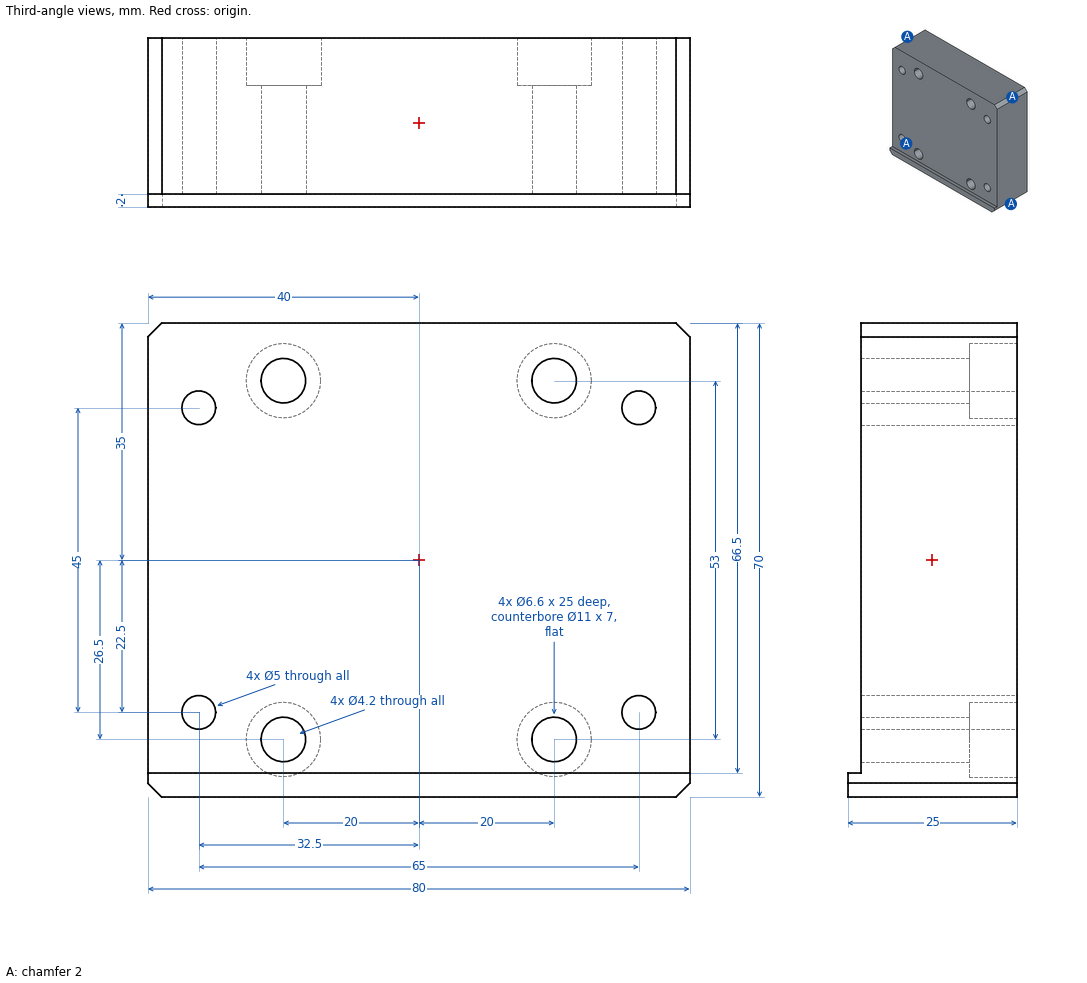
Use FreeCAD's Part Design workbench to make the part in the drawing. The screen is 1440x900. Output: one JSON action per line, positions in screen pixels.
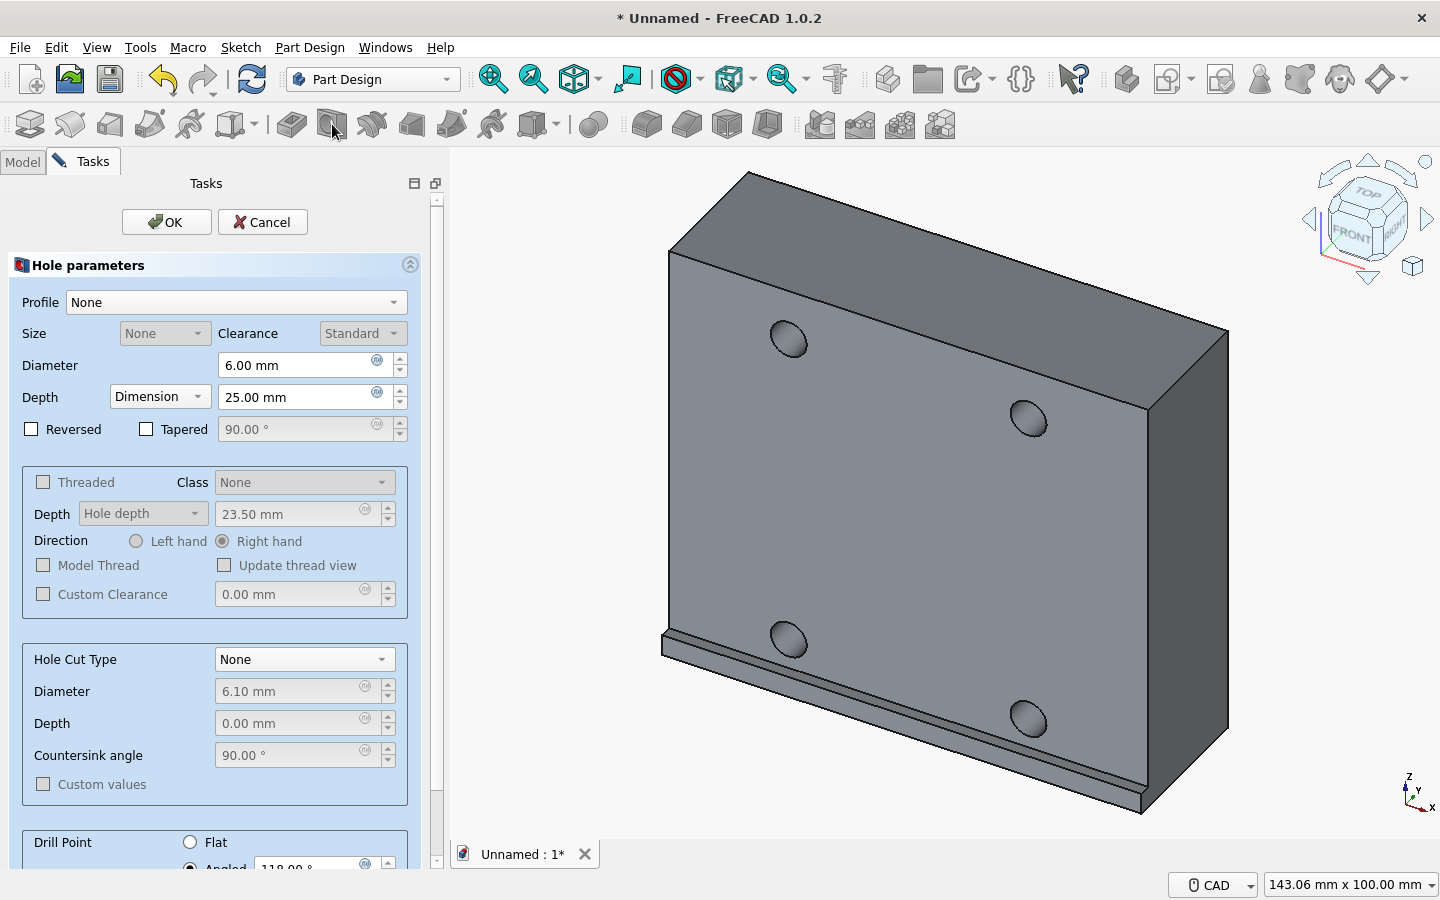
{"action": "triple_click", "coordinate": [305, 365]}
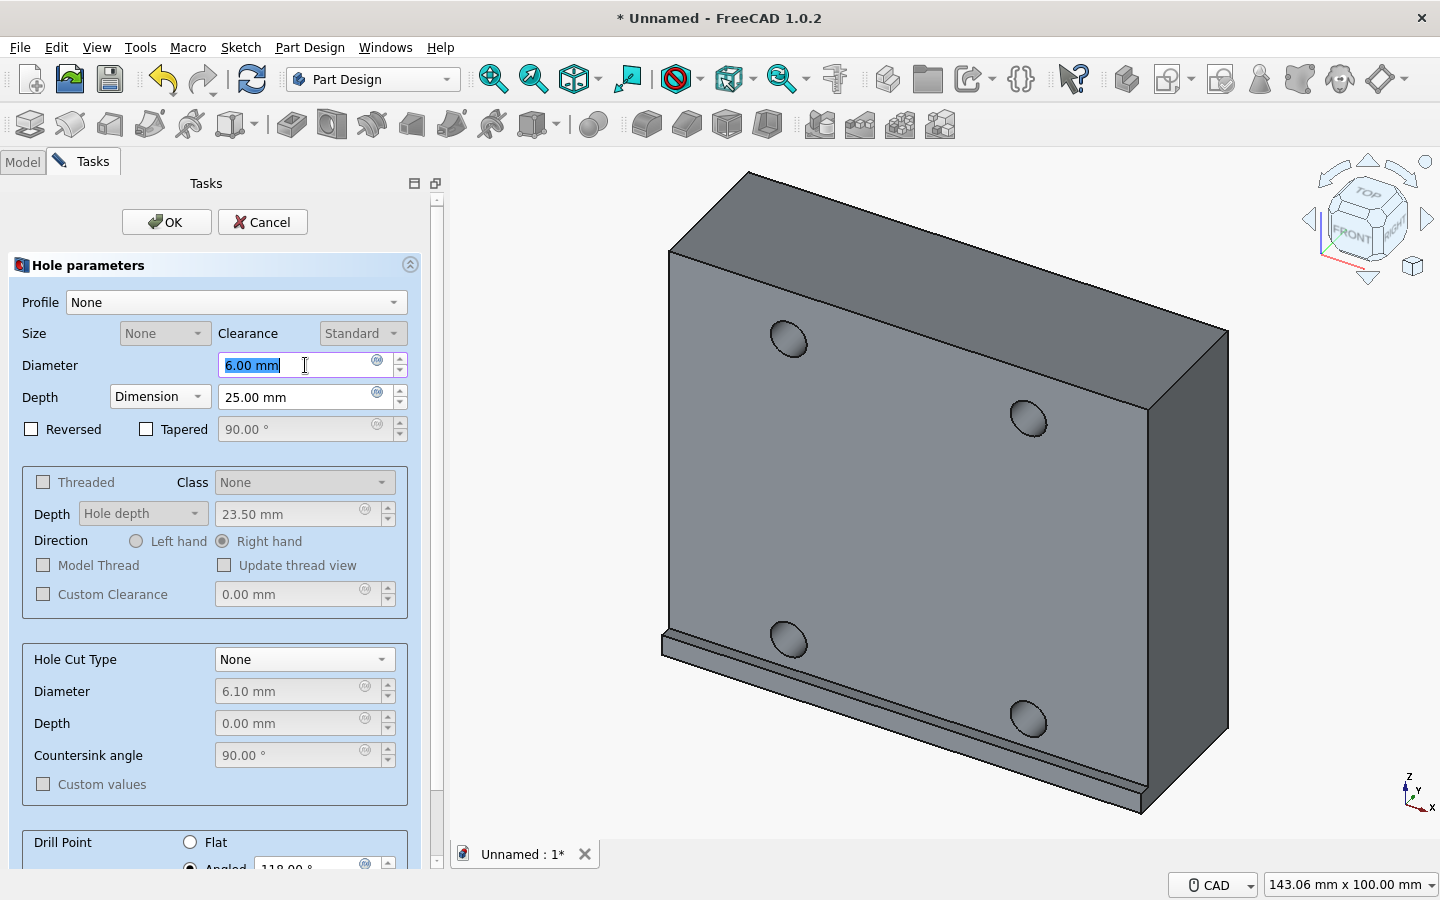
{"action": "type", "text": "4.2"}
{"action": "key", "text": "Tab"}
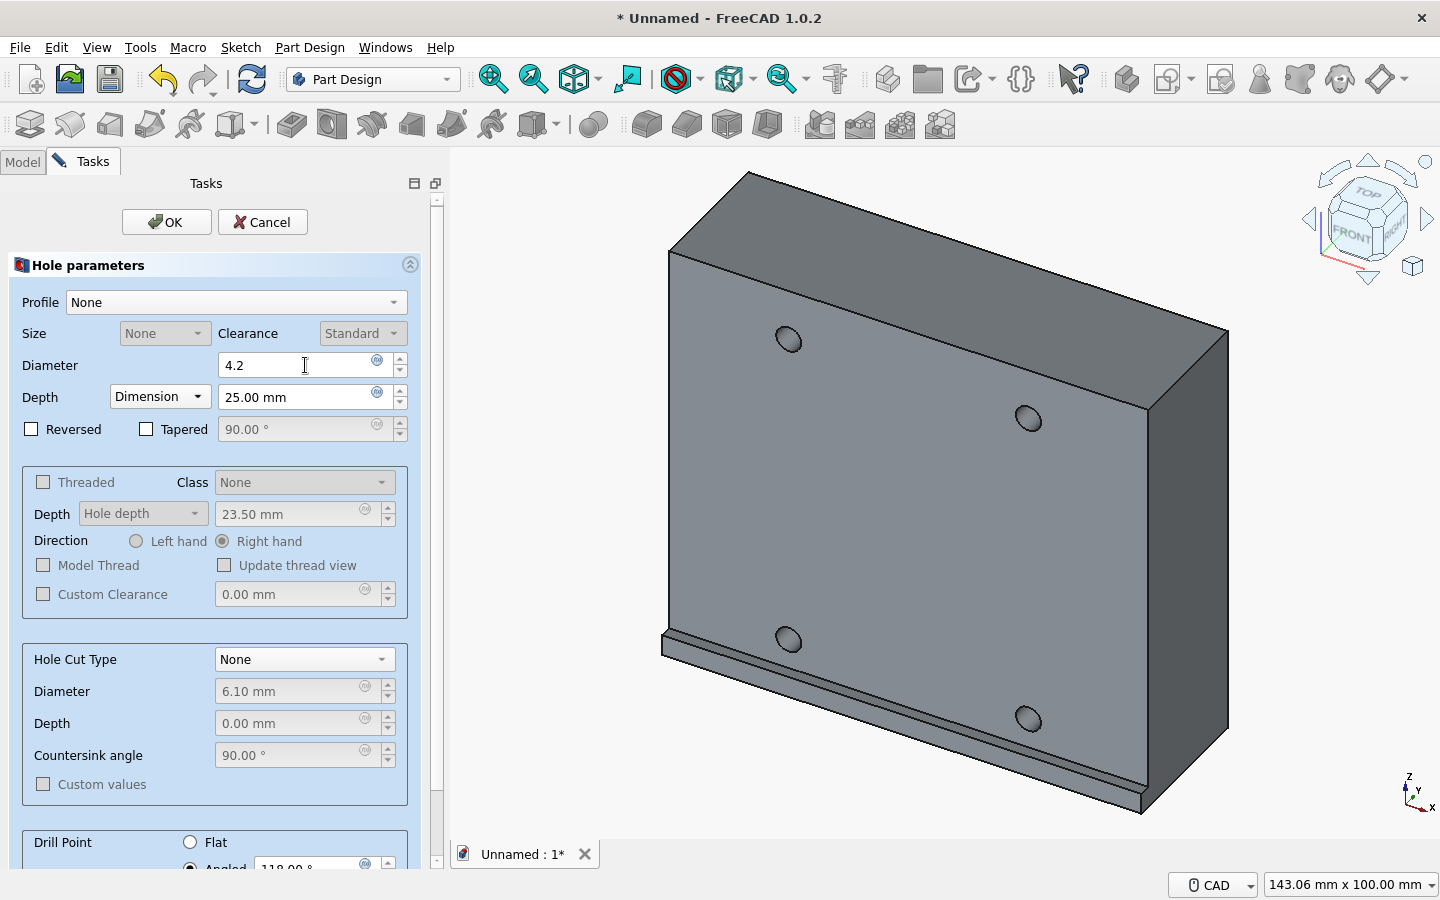
{"action": "left_click", "coordinate": [161, 396]}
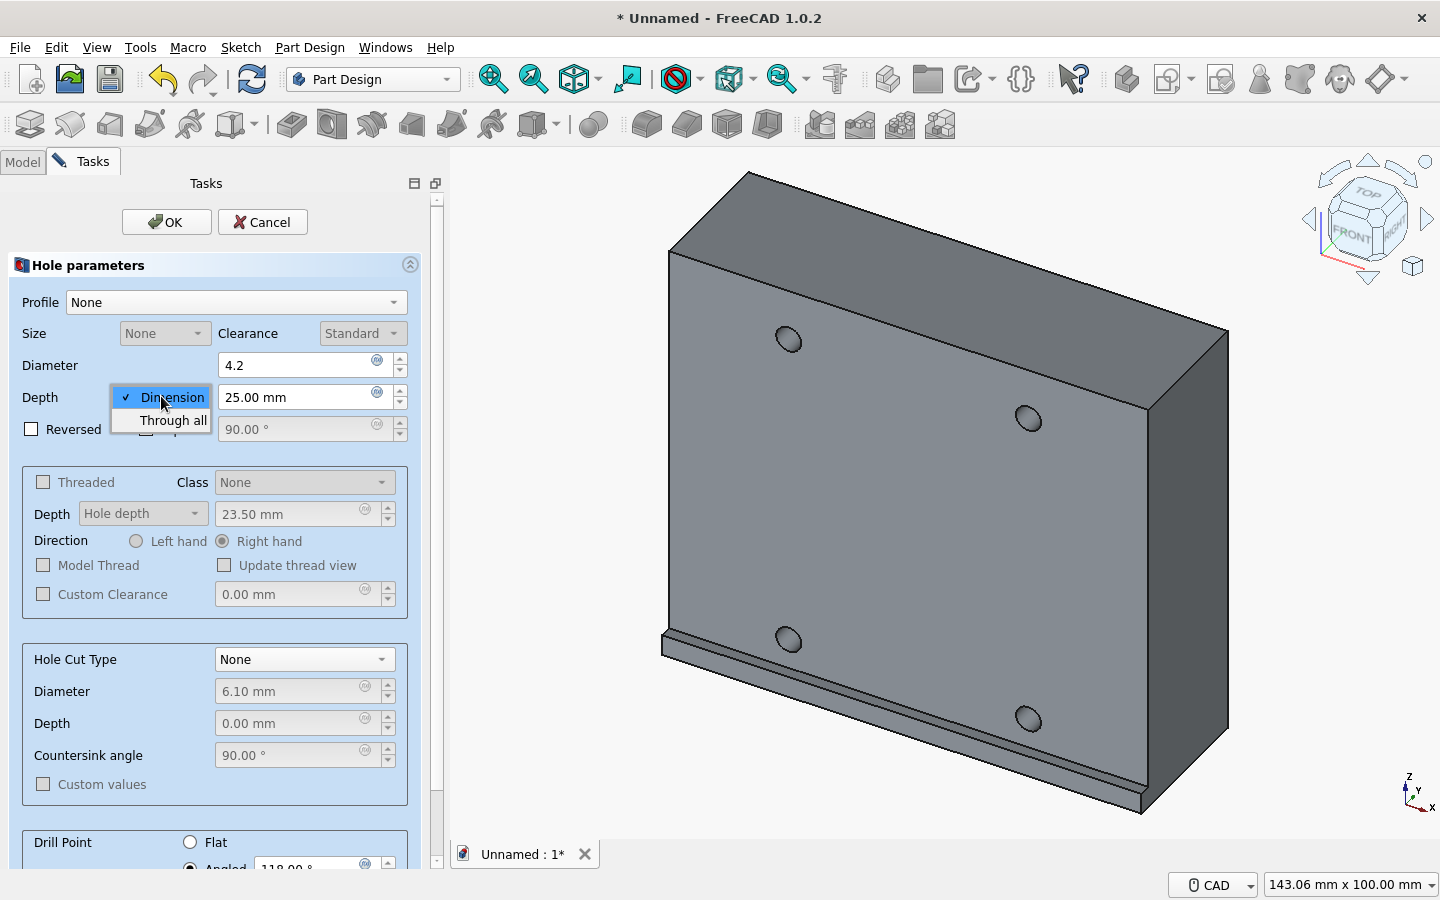
{"action": "left_click", "coordinate": [160, 420]}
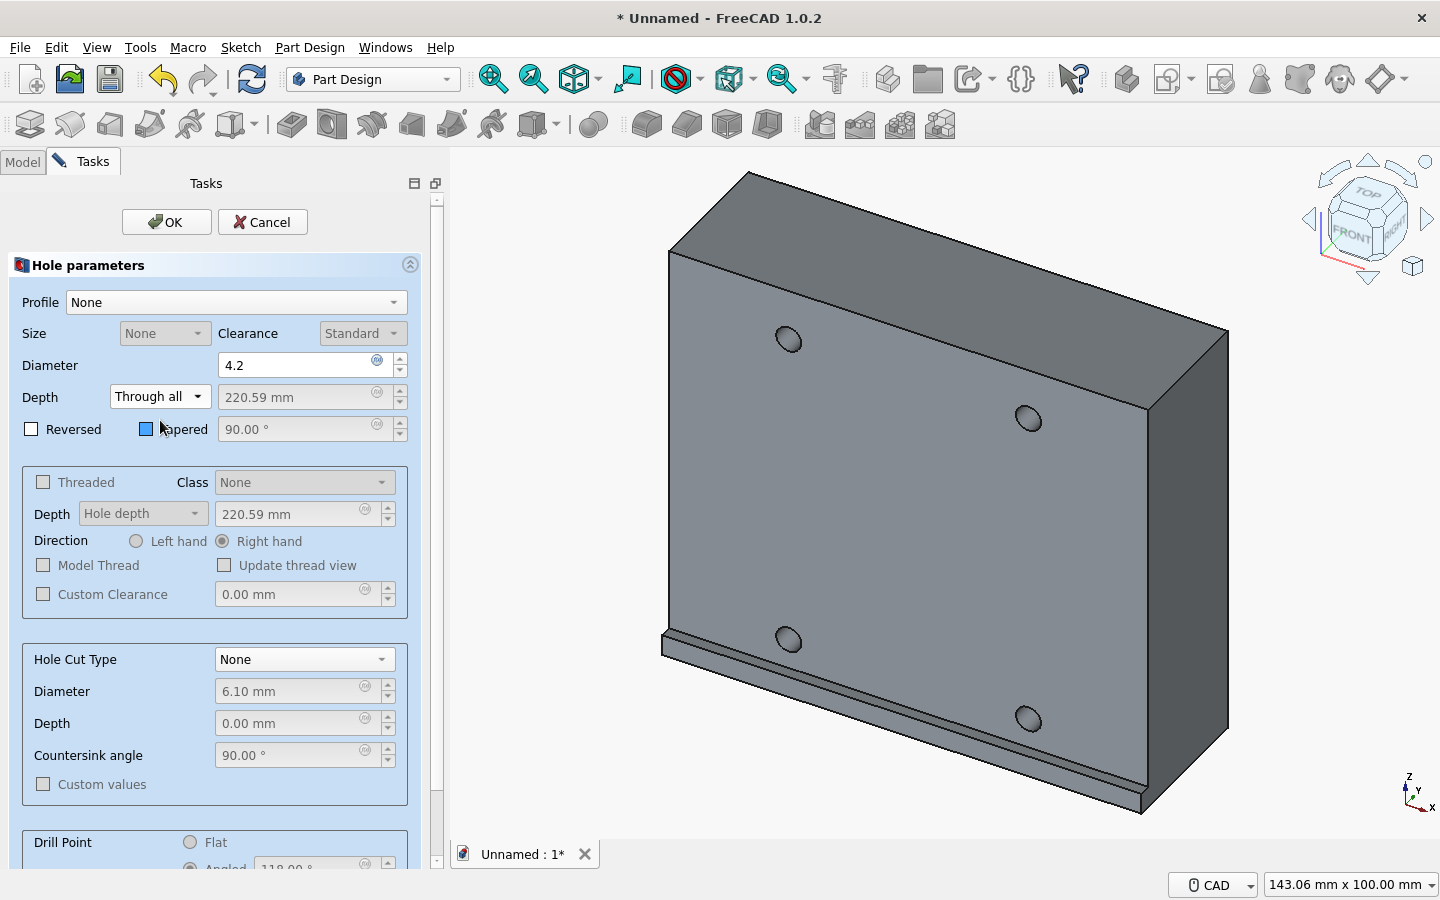
{"action": "left_click", "coordinate": [167, 222]}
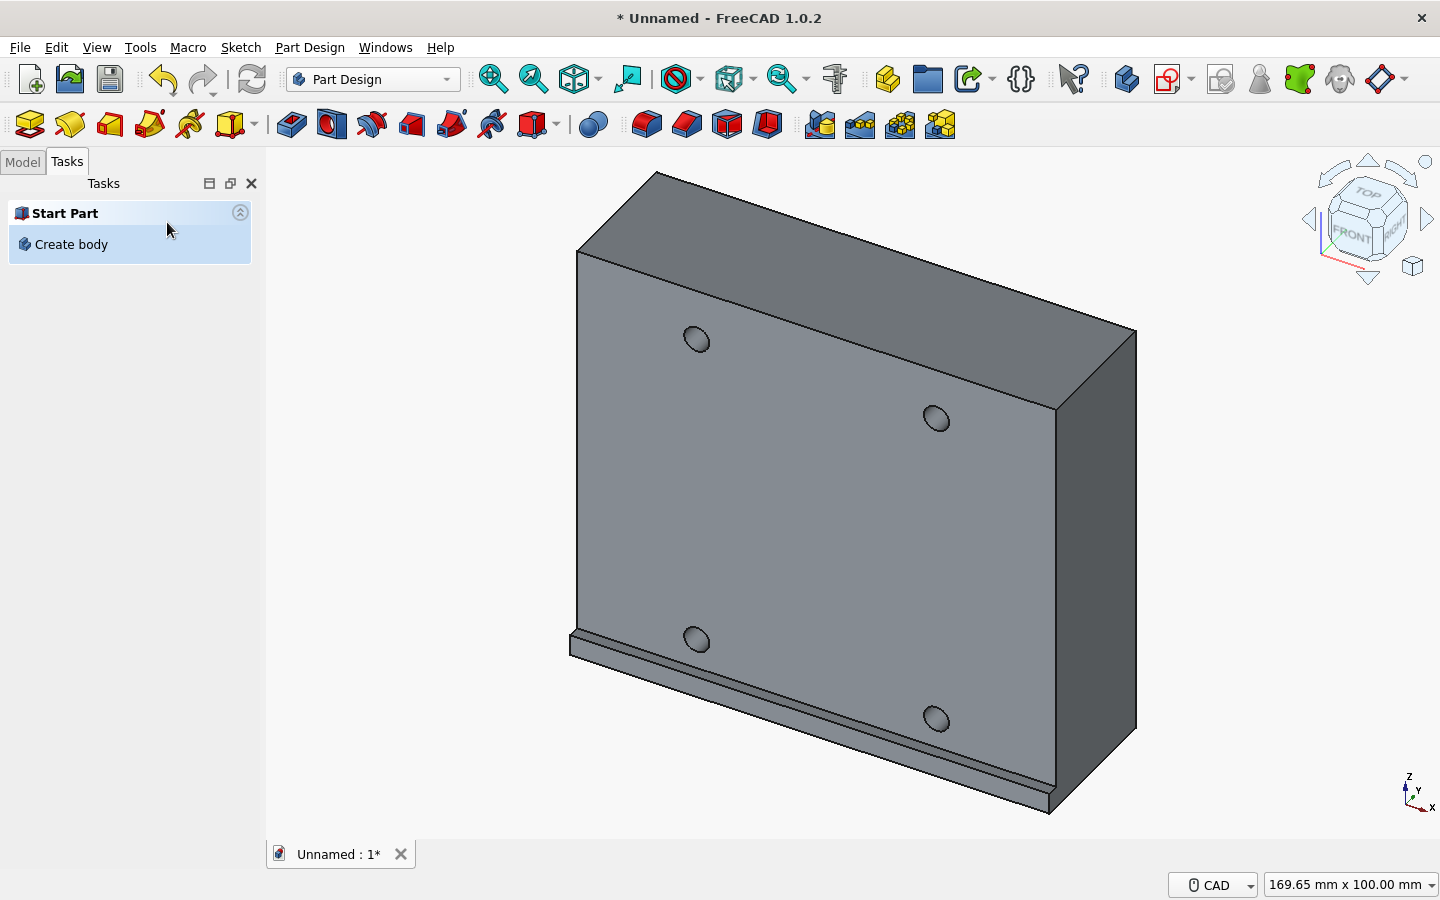
{"action": "left_click", "coordinate": [817, 518]}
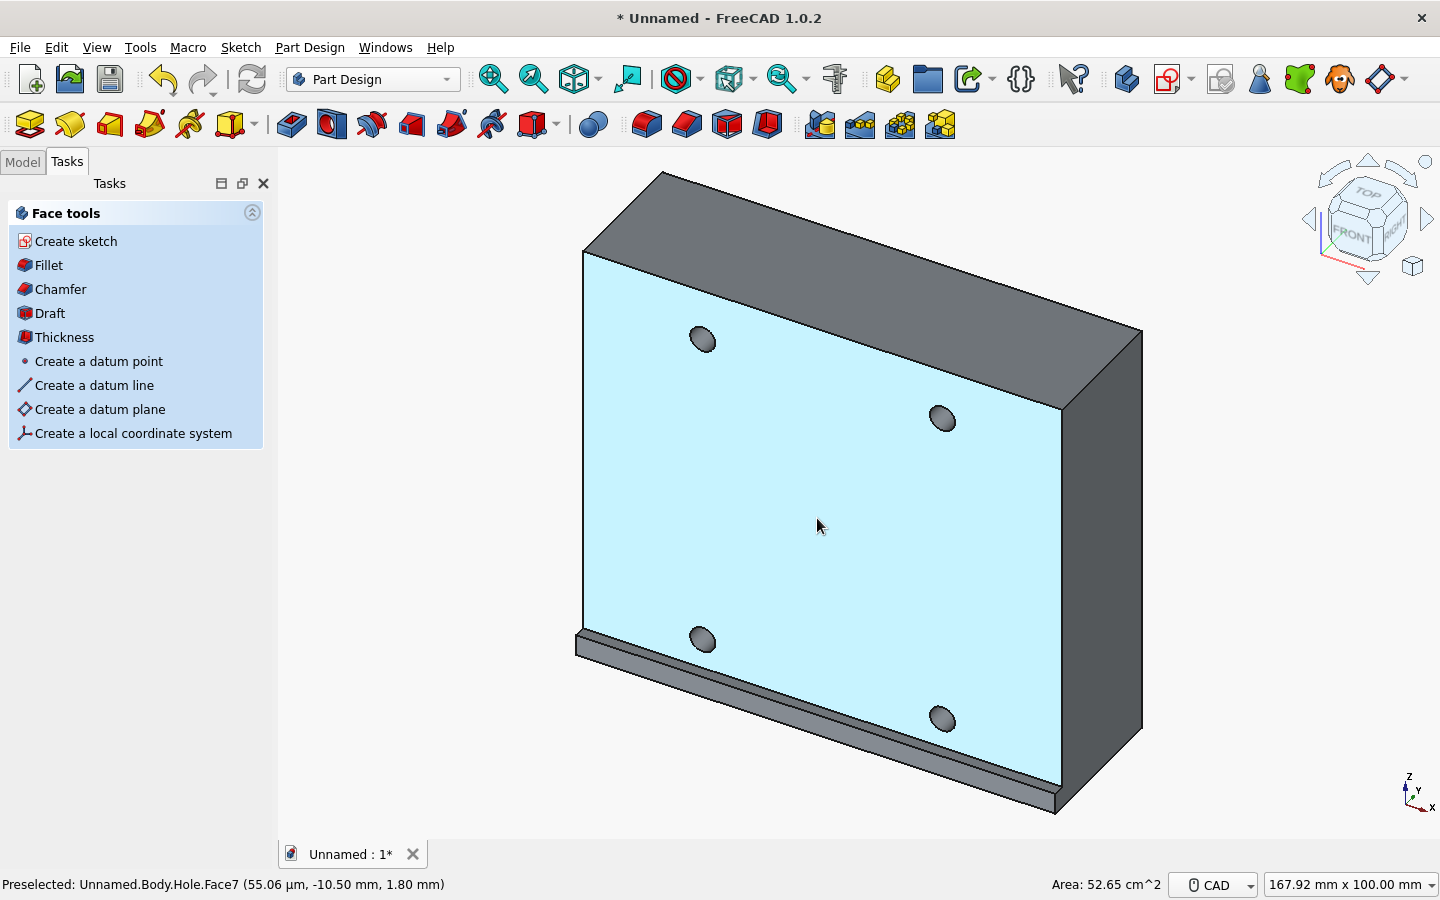
{"action": "left_click", "coordinate": [1168, 80]}